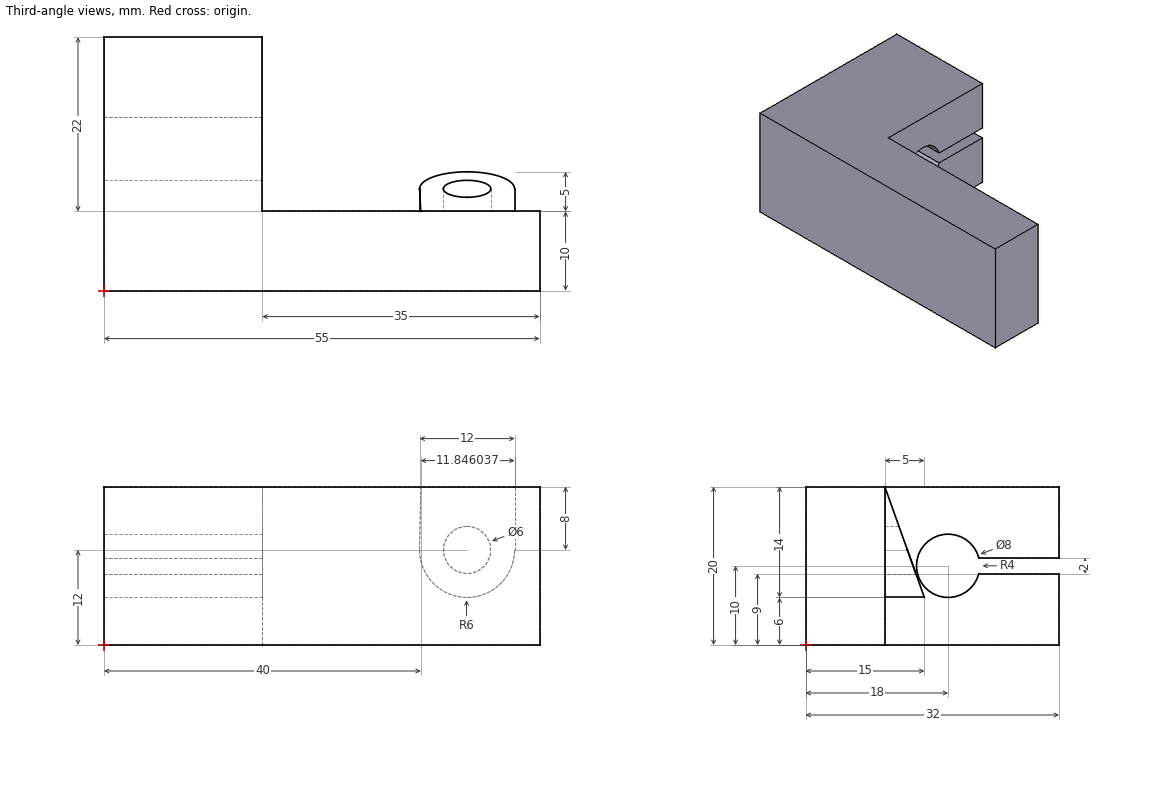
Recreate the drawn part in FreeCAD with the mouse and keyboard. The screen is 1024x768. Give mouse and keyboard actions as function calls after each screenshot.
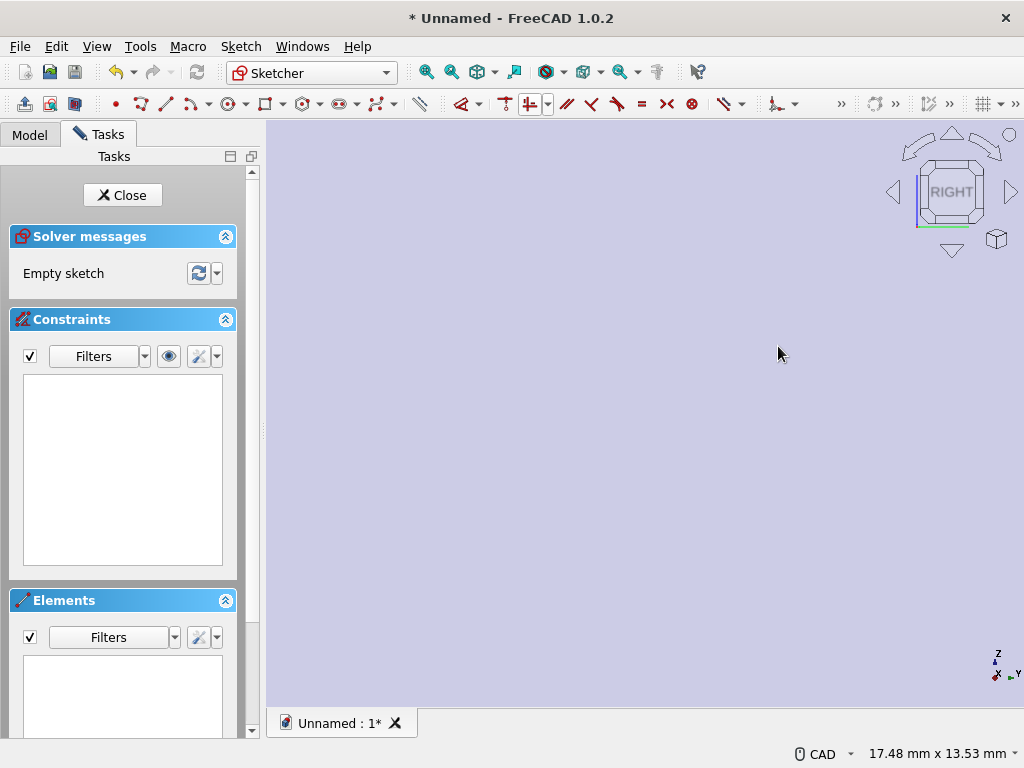
click(228, 104)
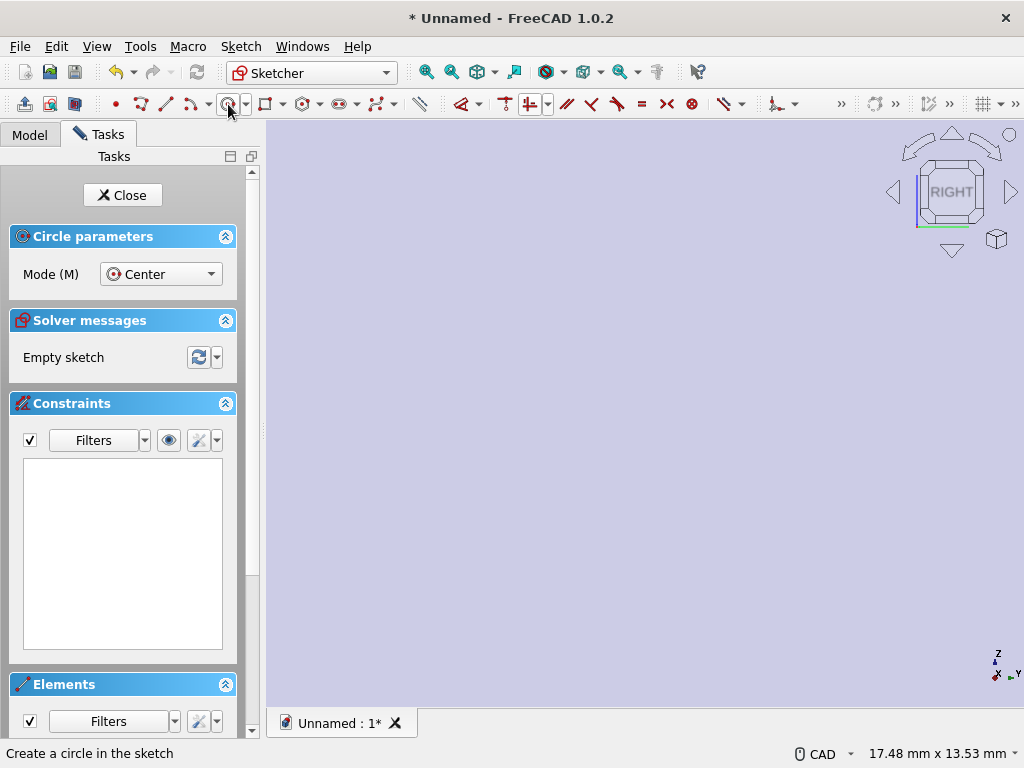
click(572, 409)
move(694, 286)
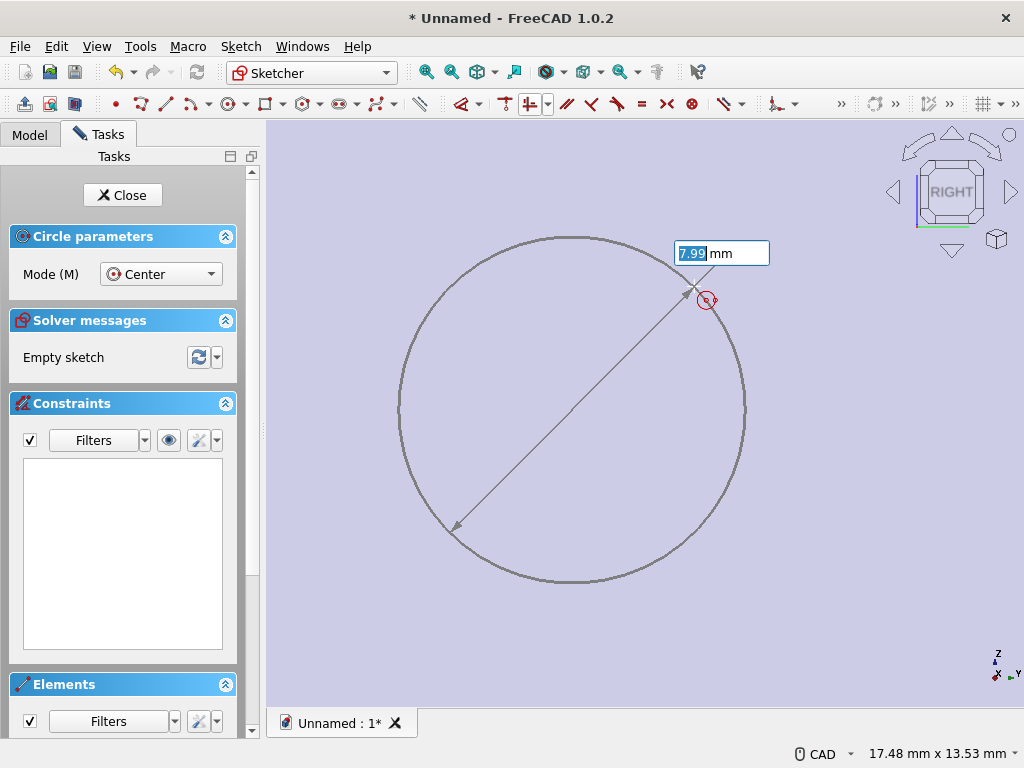
text(8)
key(Return)
key(Escape)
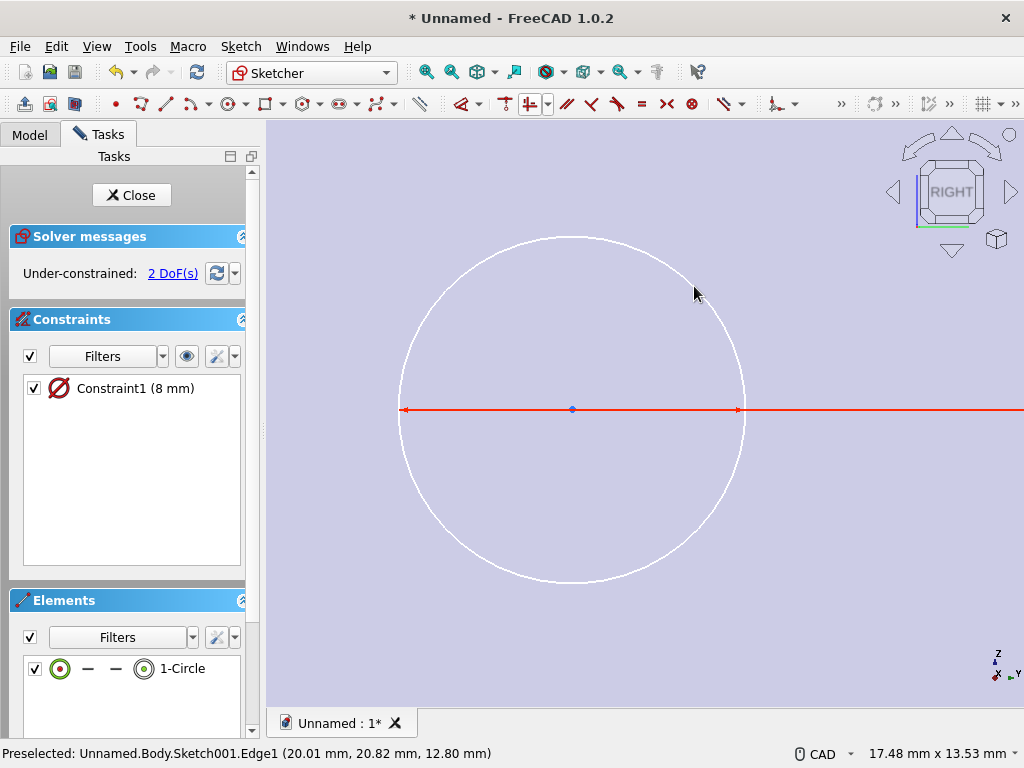
key(d)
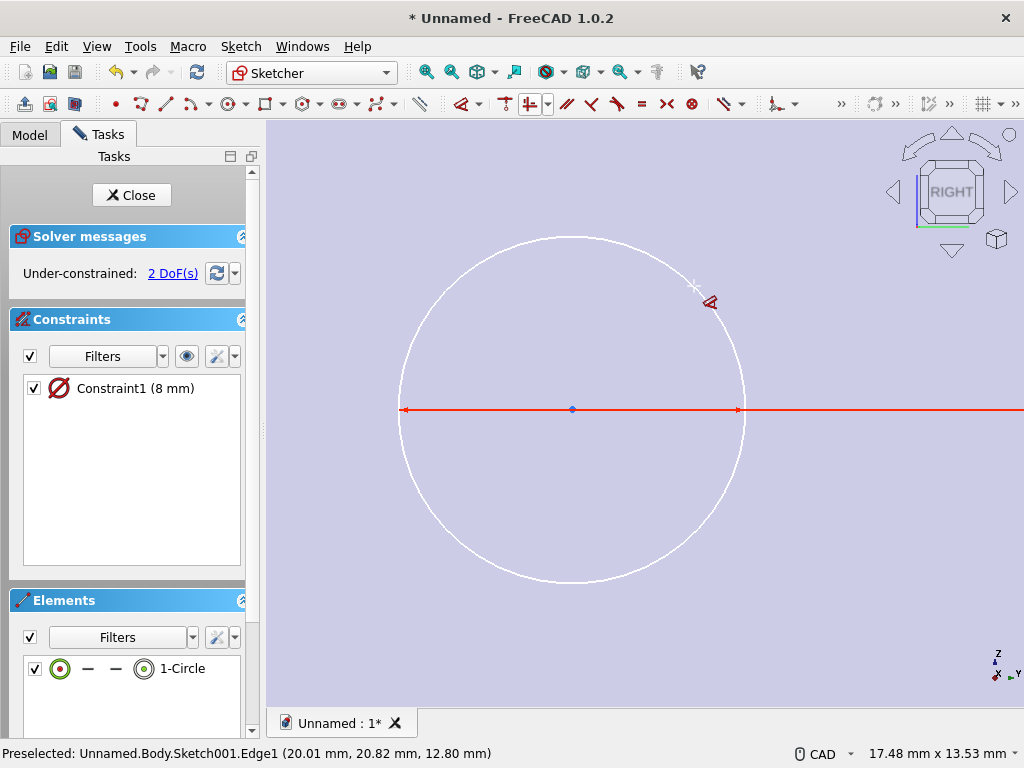
click(572, 410)
click(433, 376)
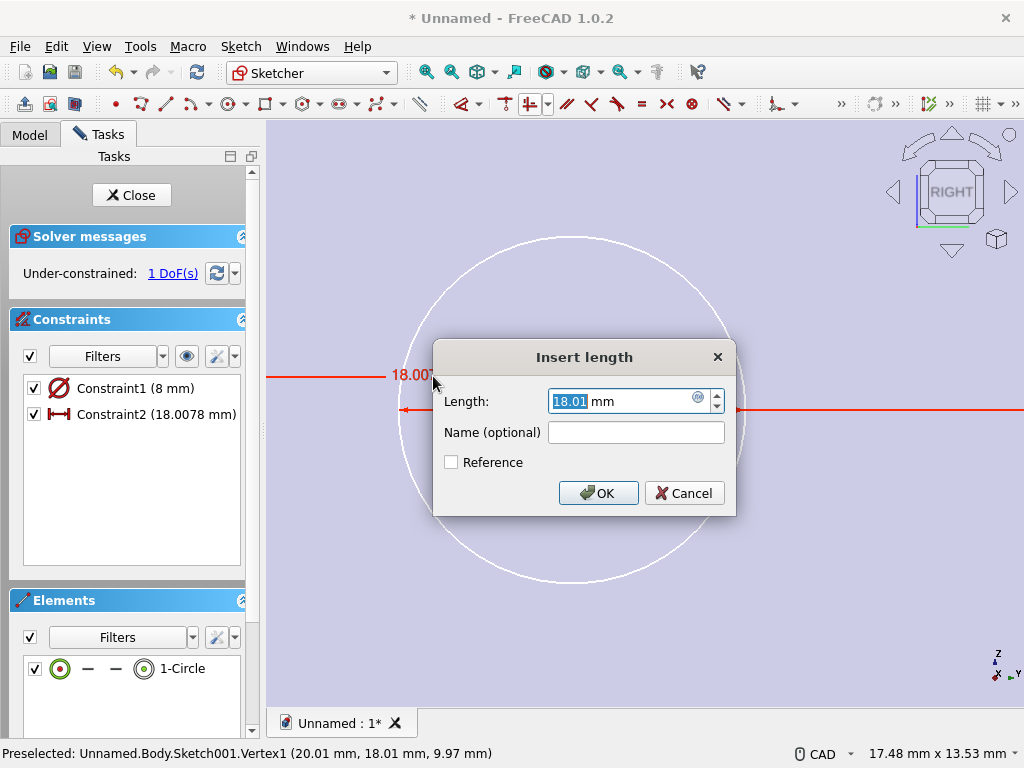
text(18)
key(Return)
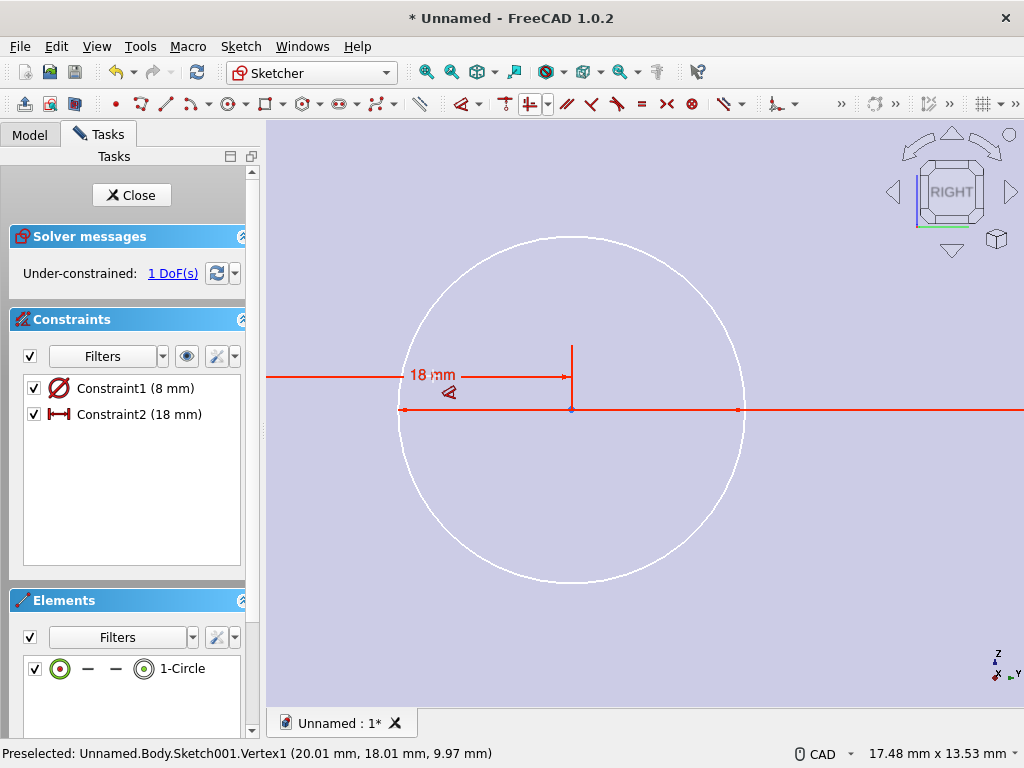
click(572, 410)
click(606, 544)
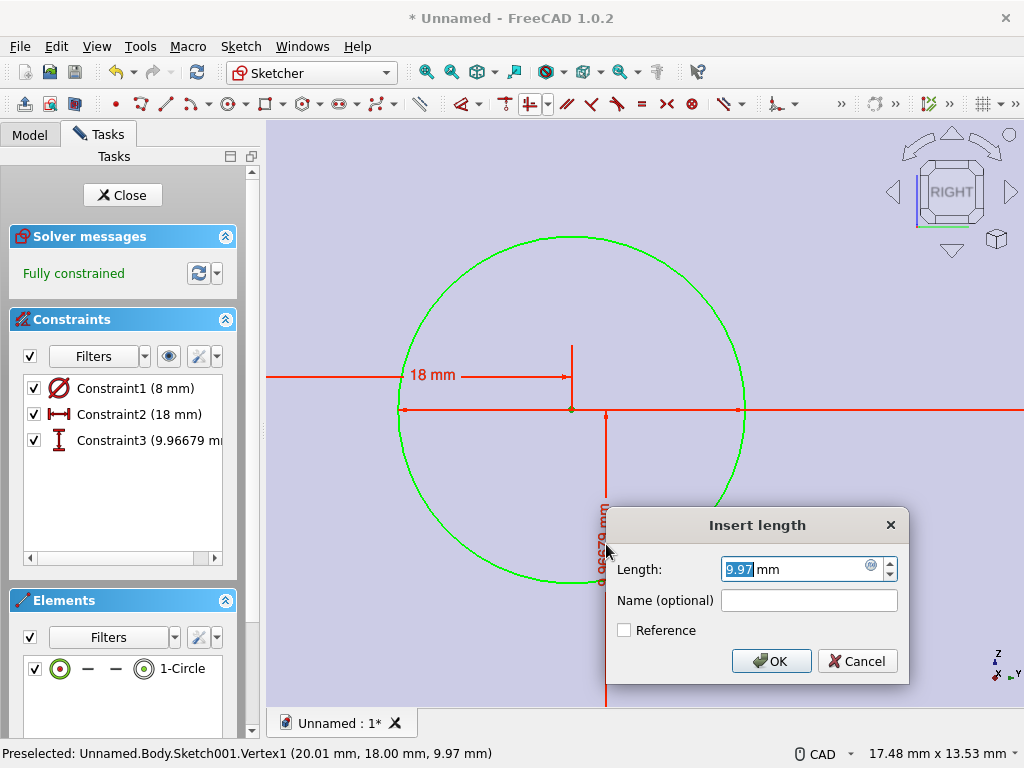
text(10)
key(Return)
key(Escape)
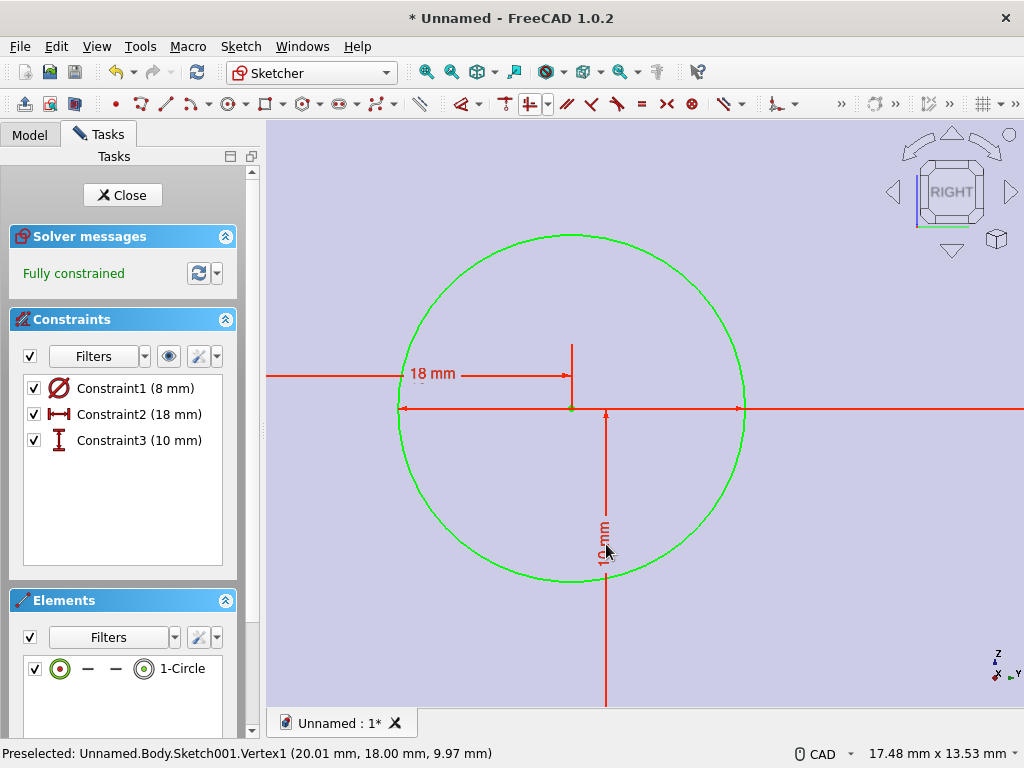
click(123, 195)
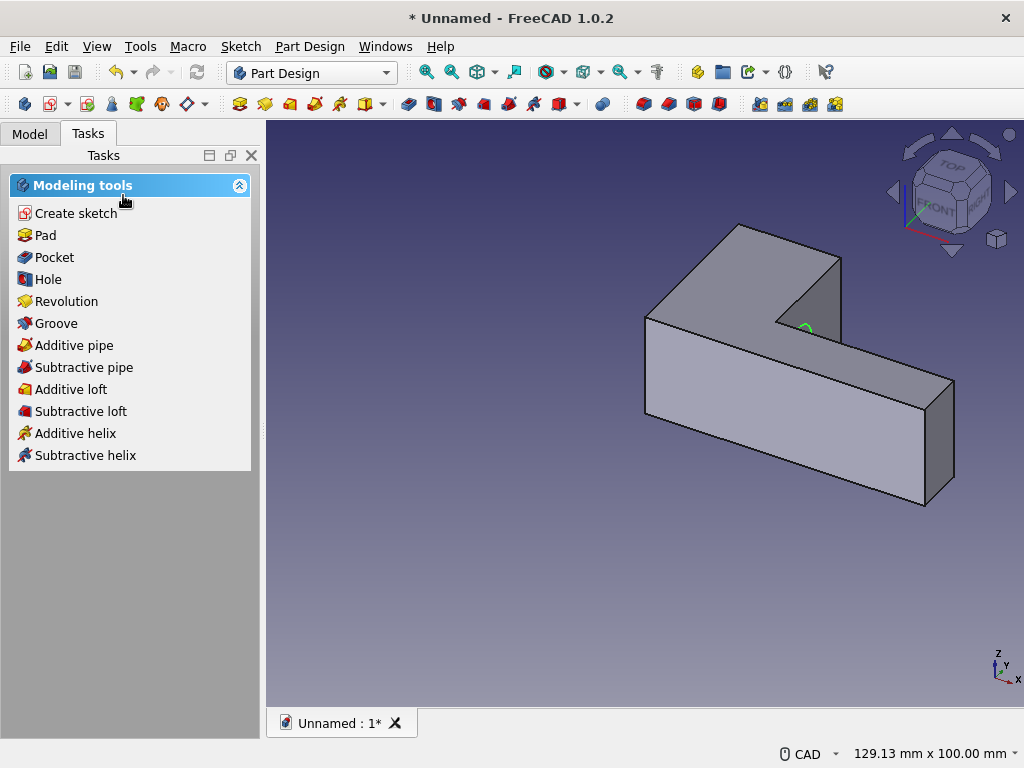
click(409, 104)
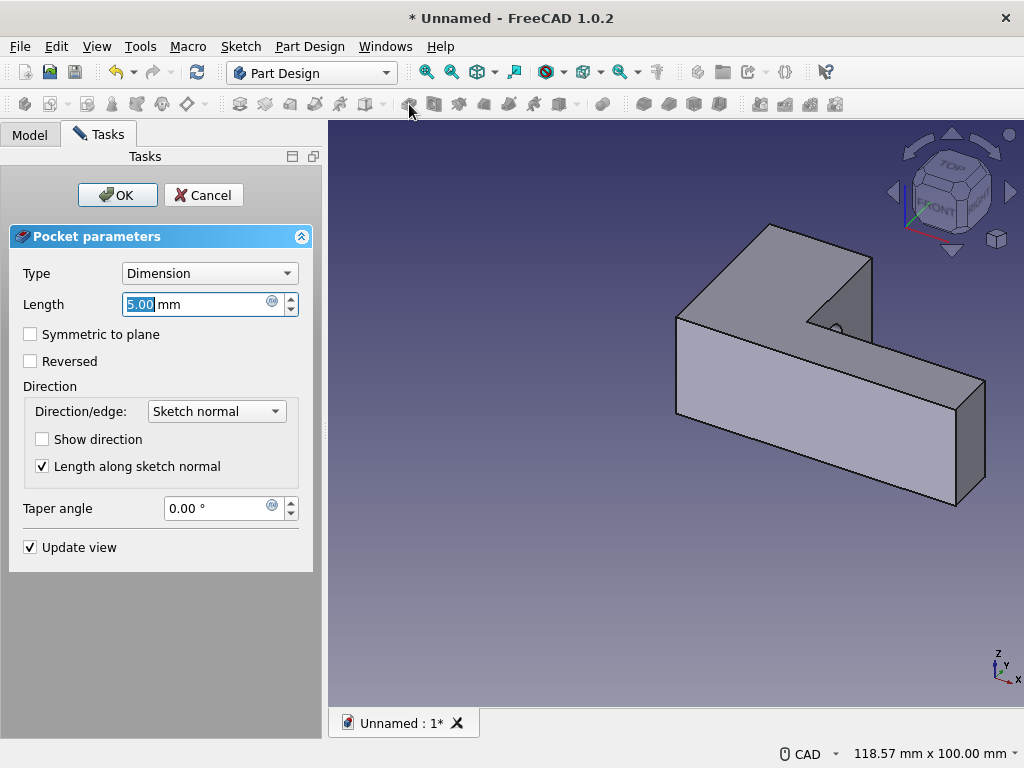
click(210, 274)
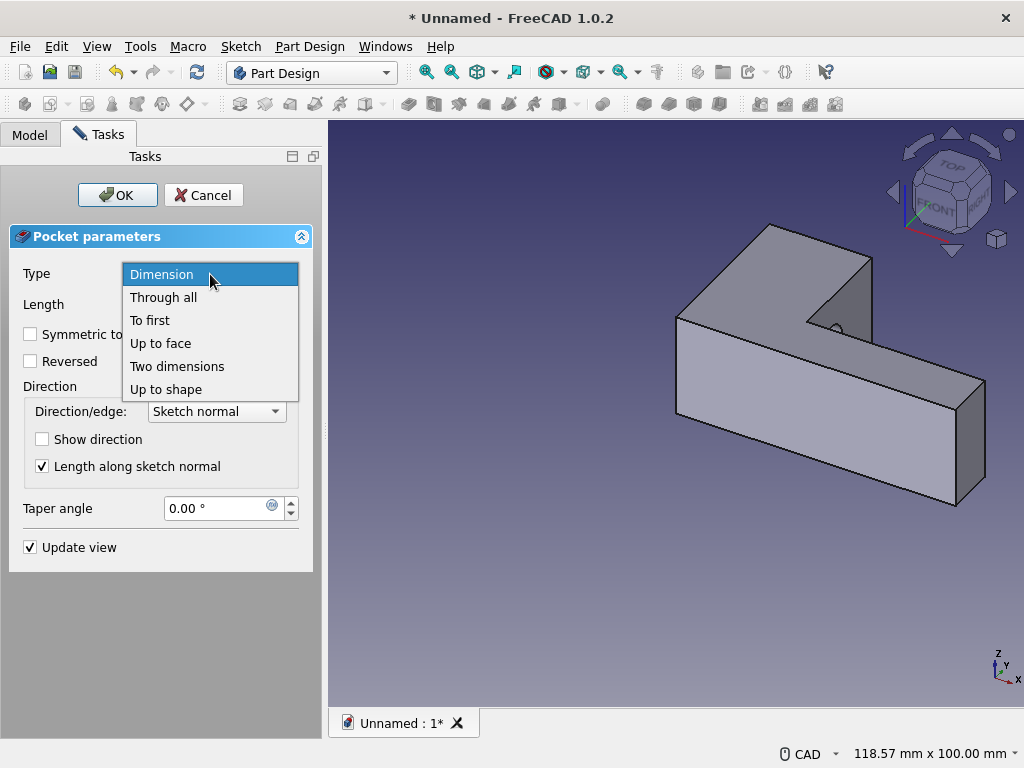
click(208, 298)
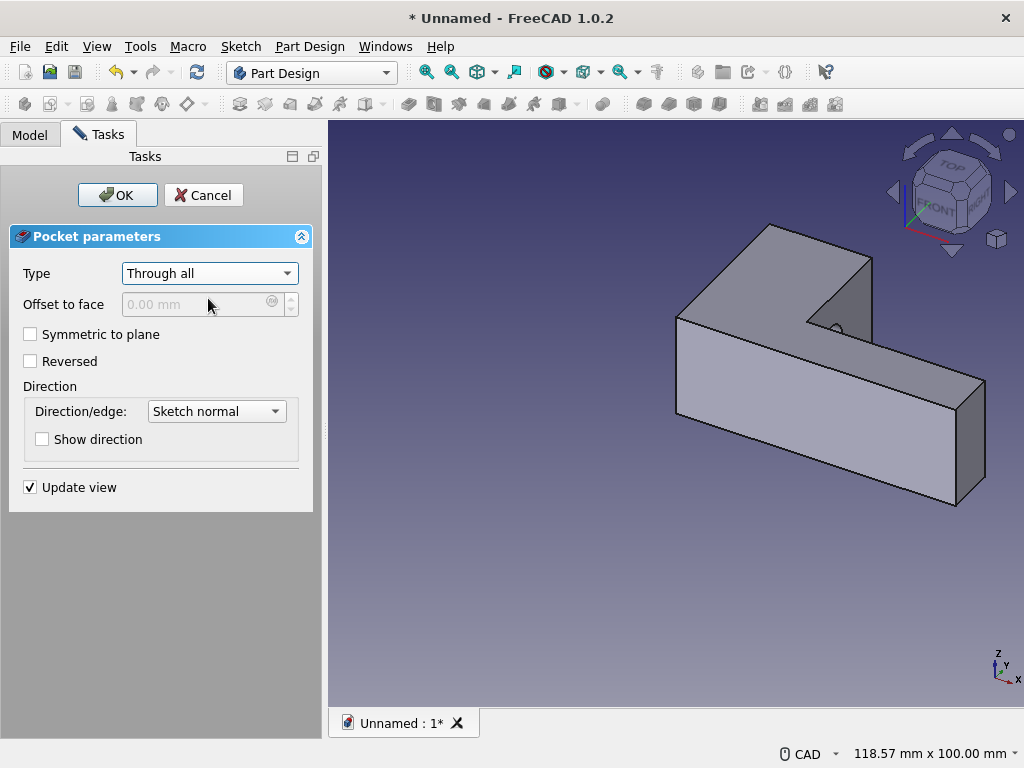
click(118, 195)